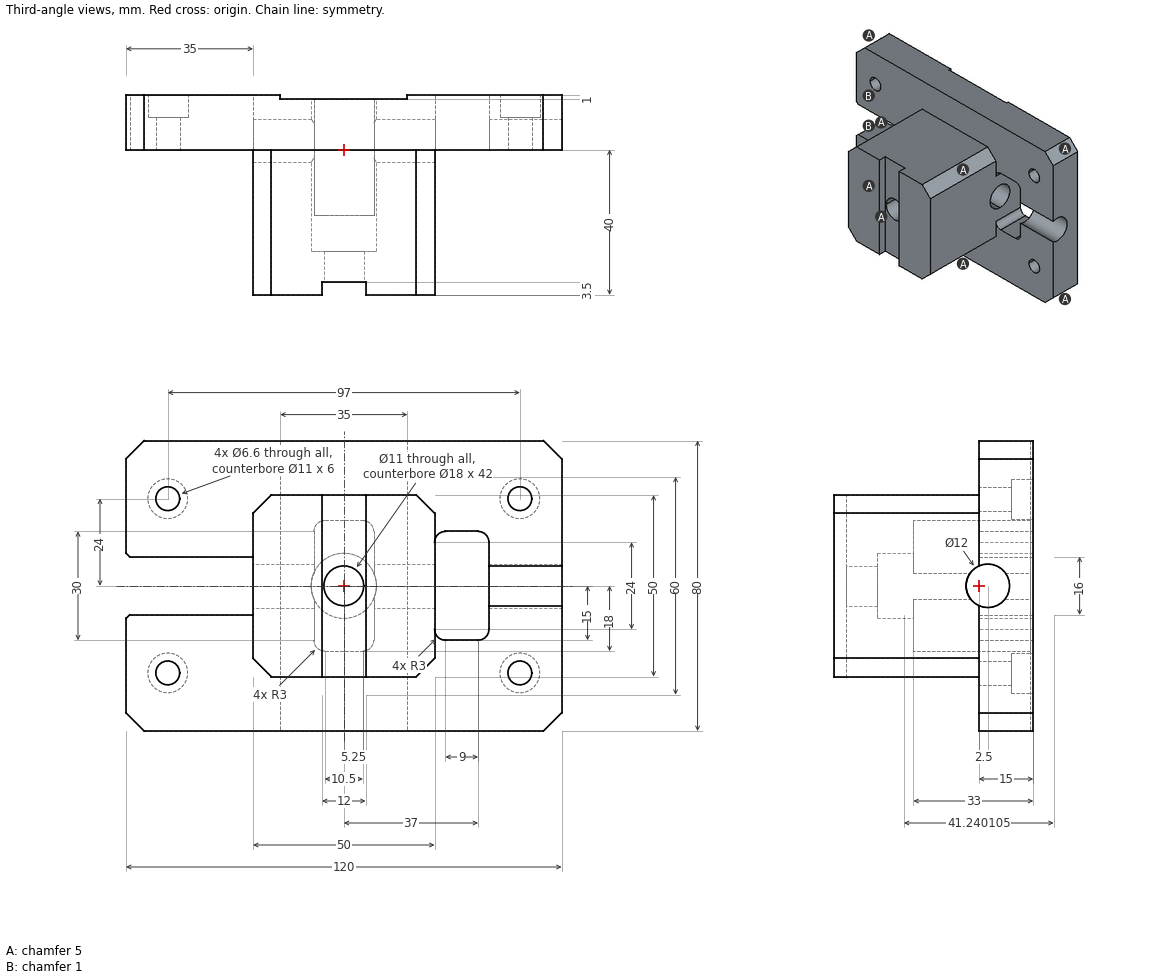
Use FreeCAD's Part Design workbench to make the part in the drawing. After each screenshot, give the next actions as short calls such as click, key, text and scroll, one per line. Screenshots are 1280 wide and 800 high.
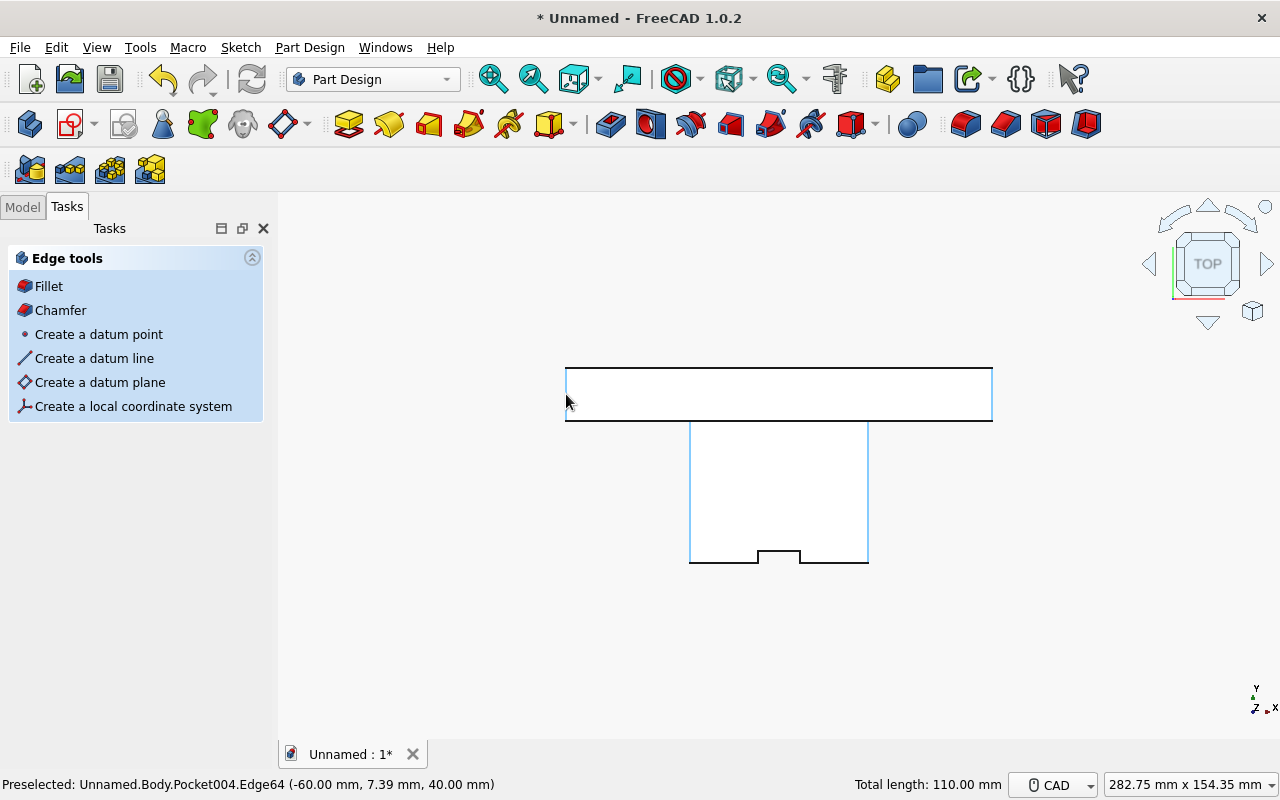
key(1)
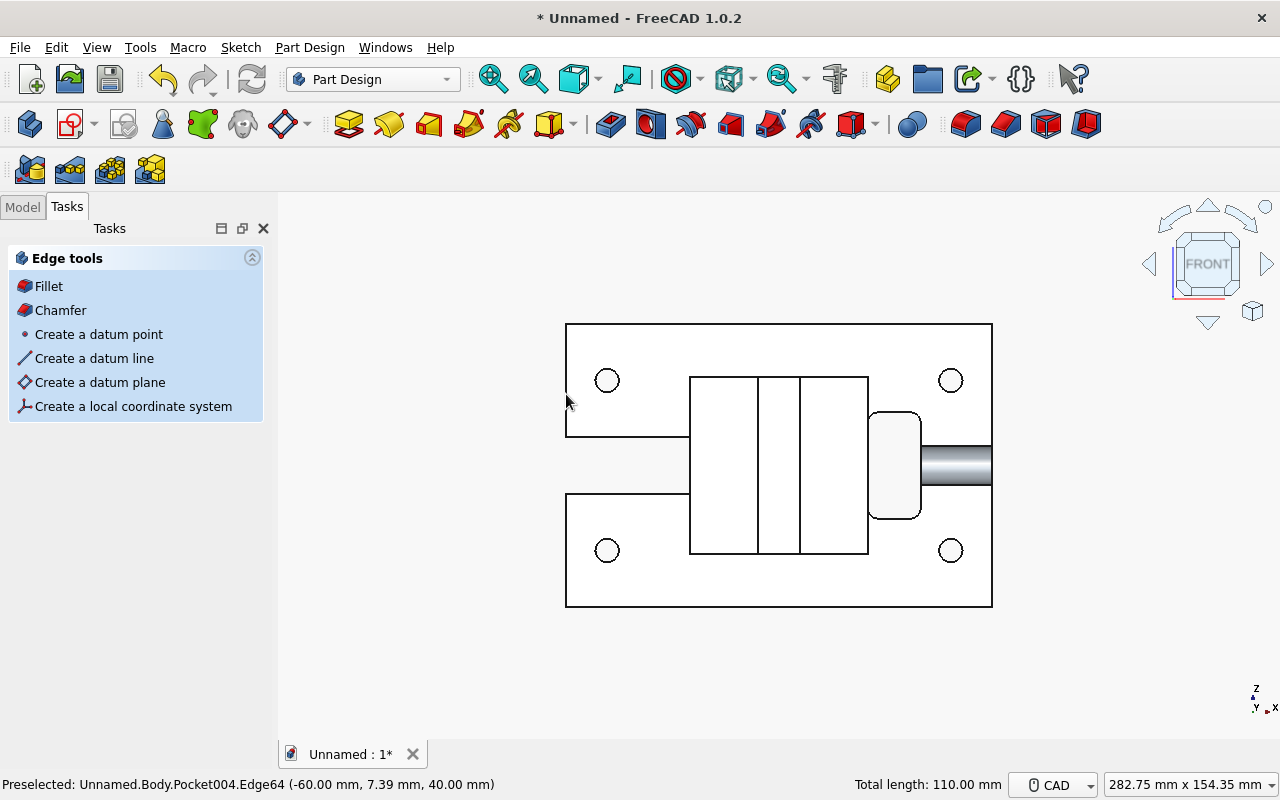
key(3)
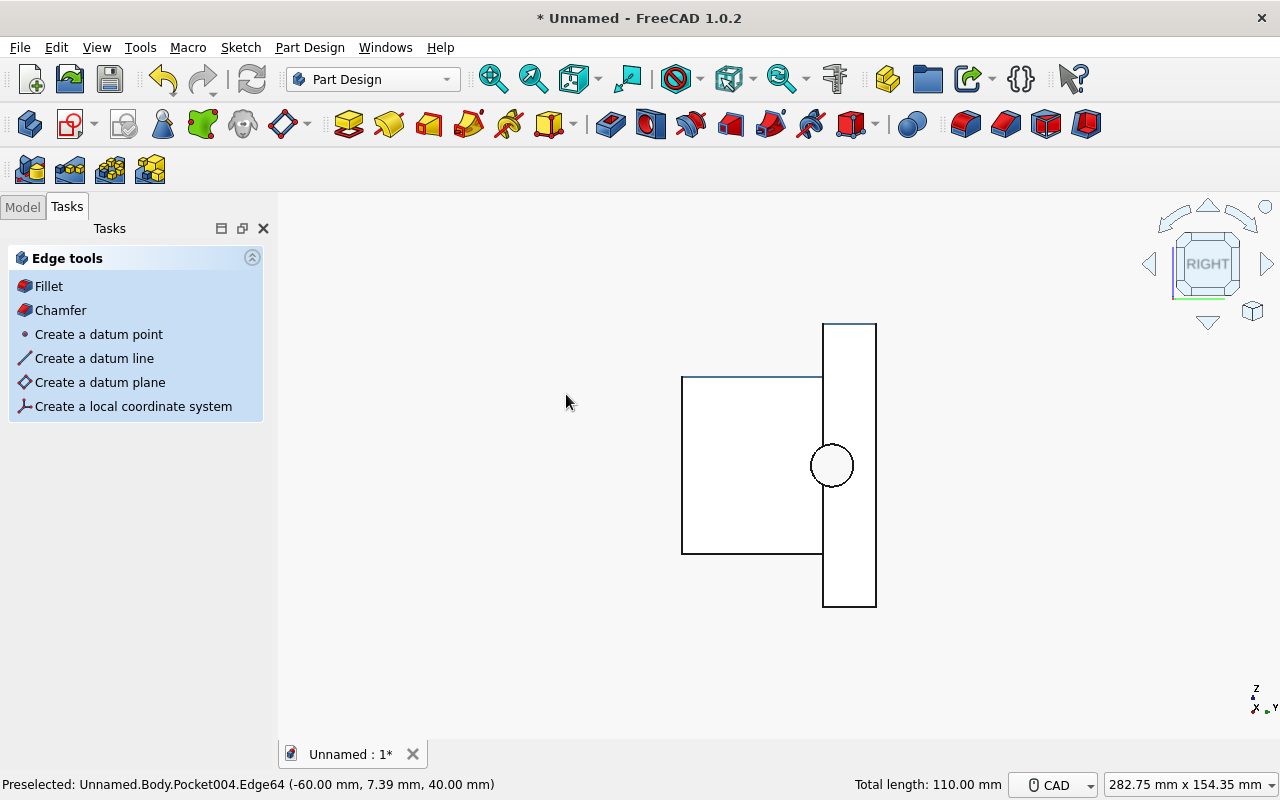
click(752, 553, ctrl)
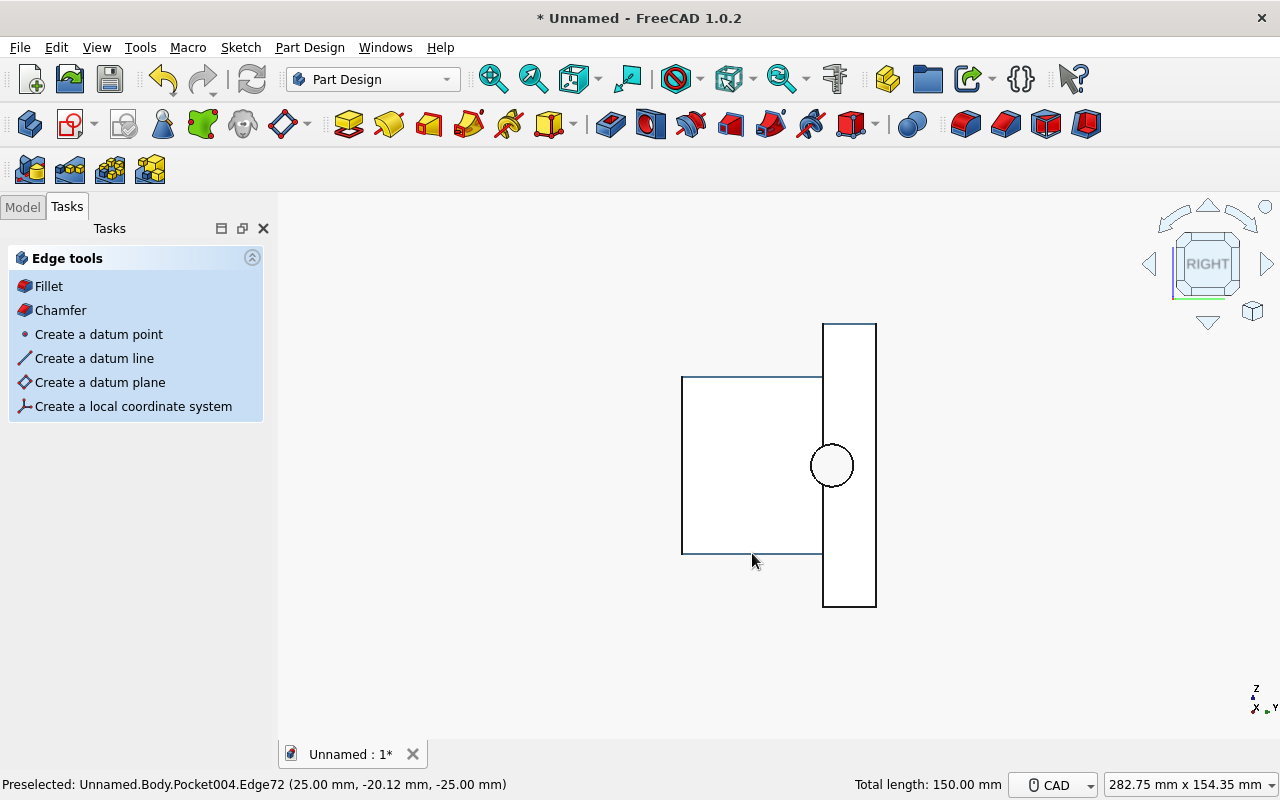
click(850, 606, ctrl)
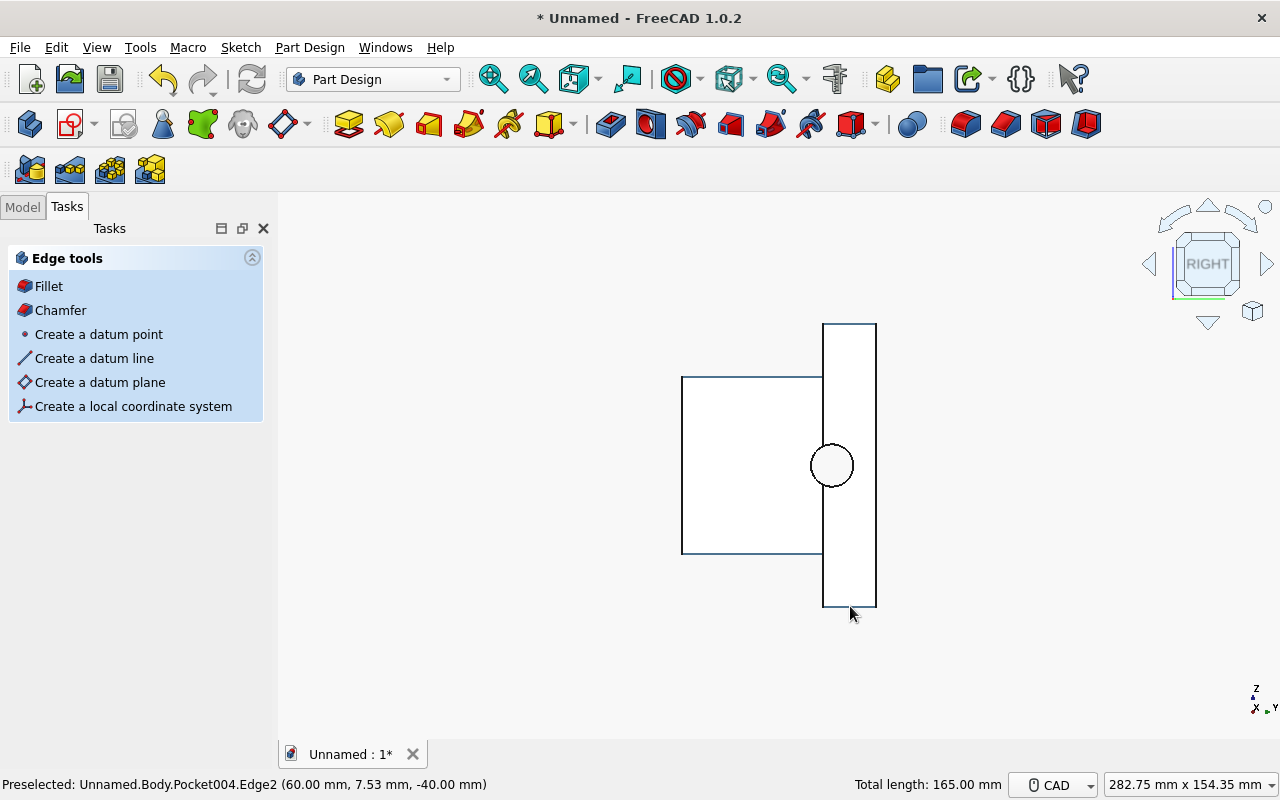
key(5)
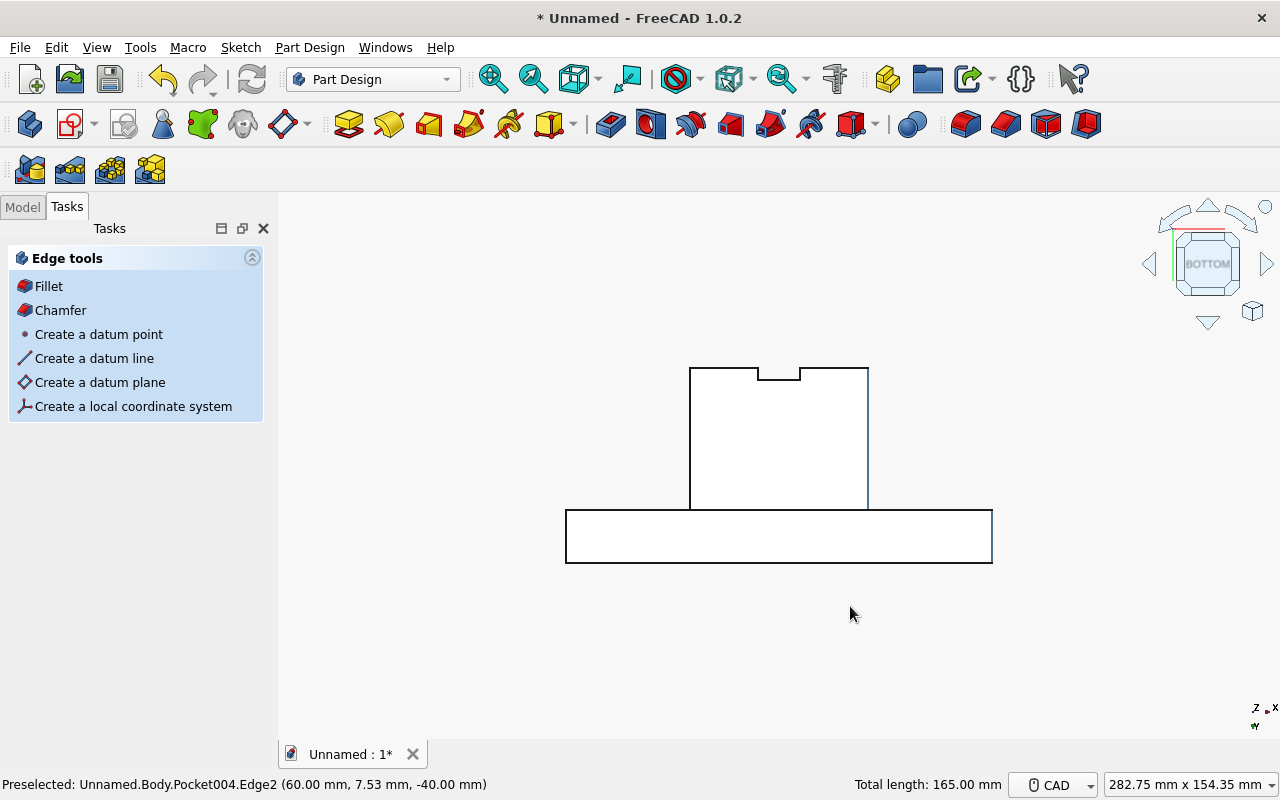
click(494, 80)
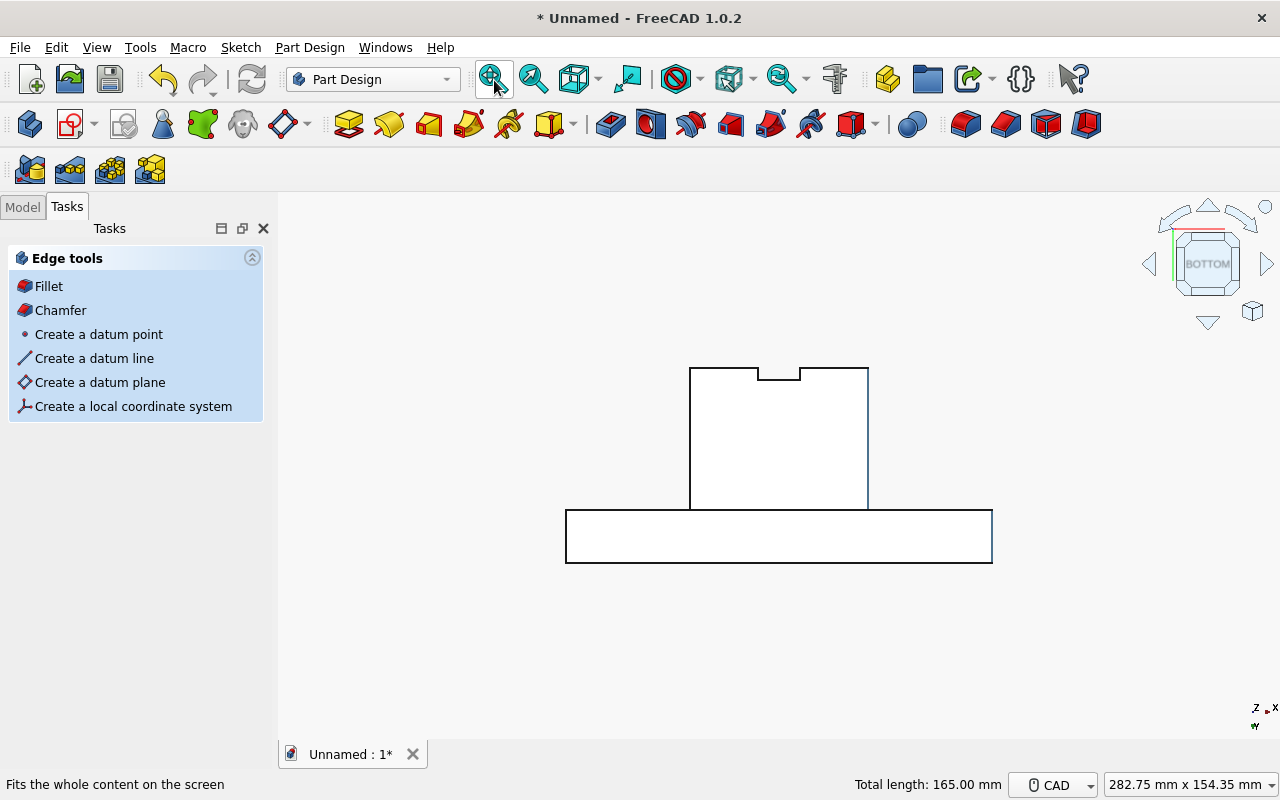
click(690, 438, ctrl)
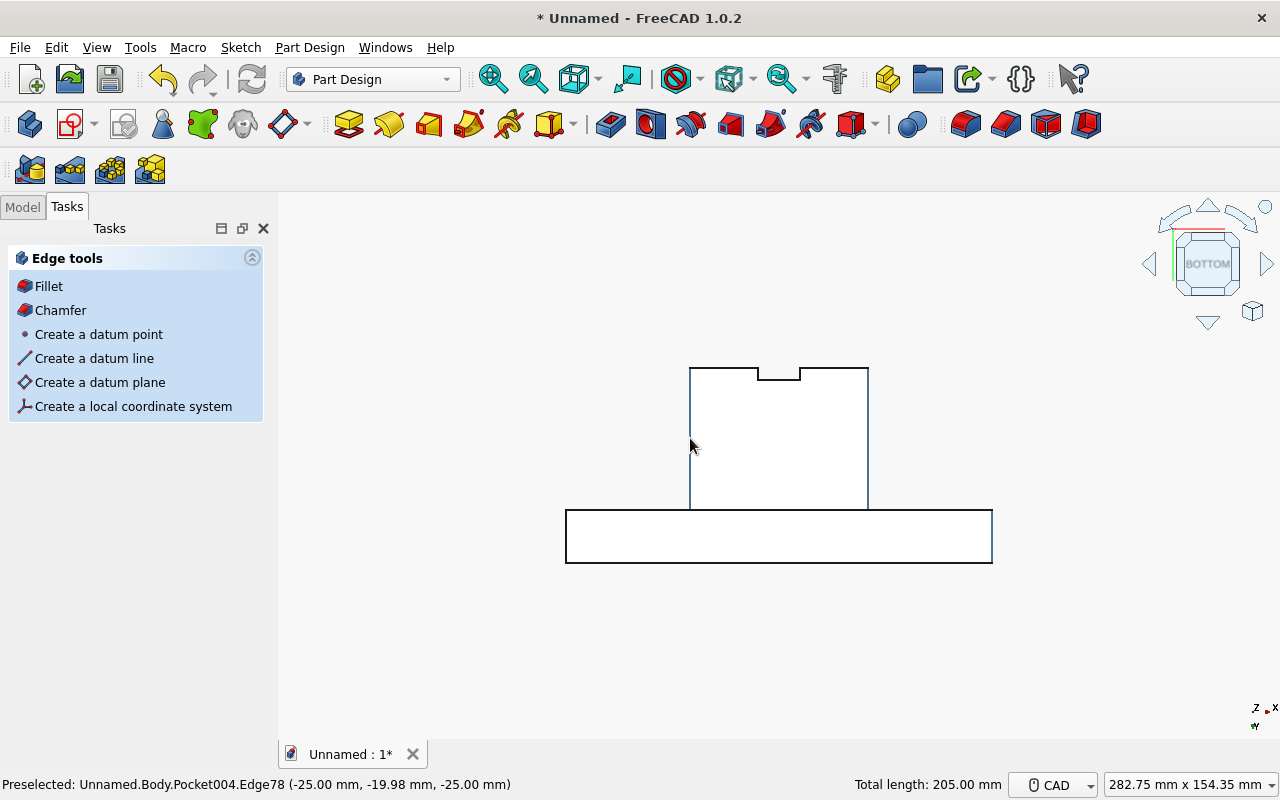
click(566, 535, ctrl)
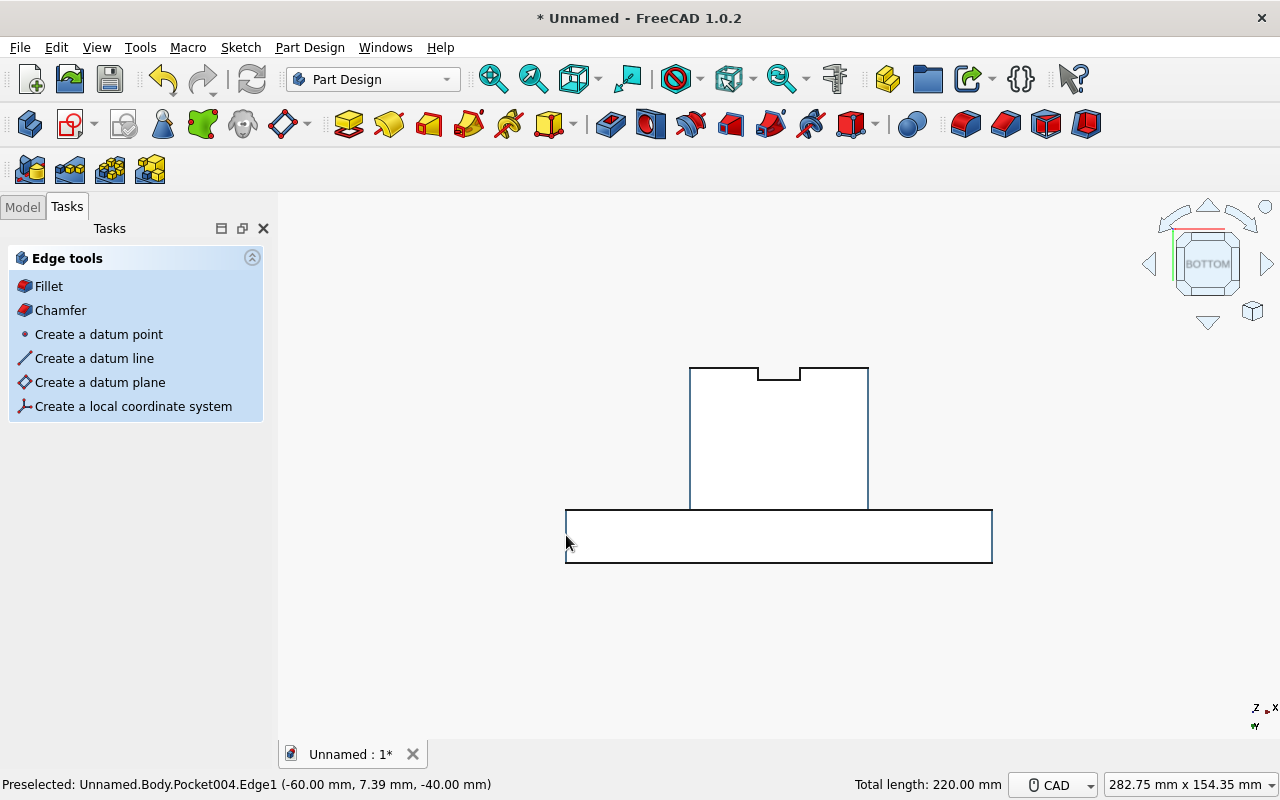
click(1006, 124)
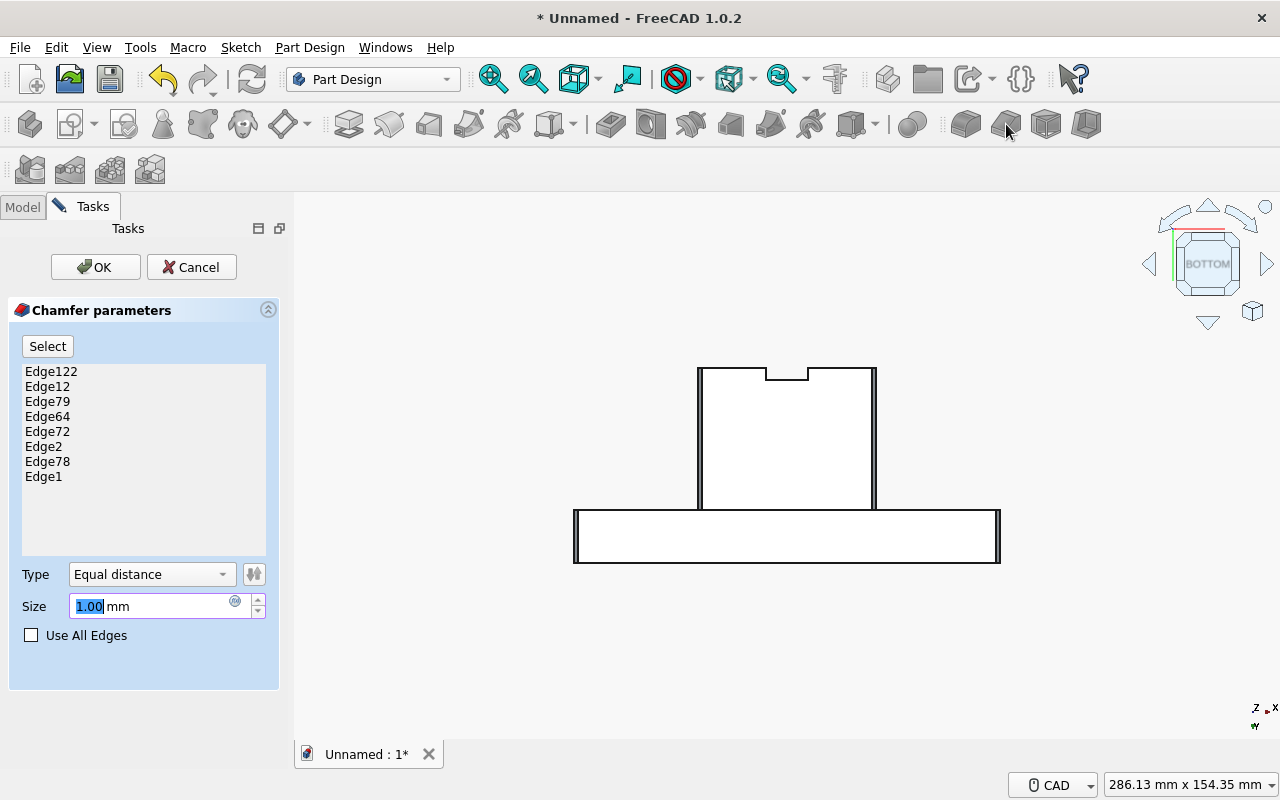
text(5)
key(Tab)